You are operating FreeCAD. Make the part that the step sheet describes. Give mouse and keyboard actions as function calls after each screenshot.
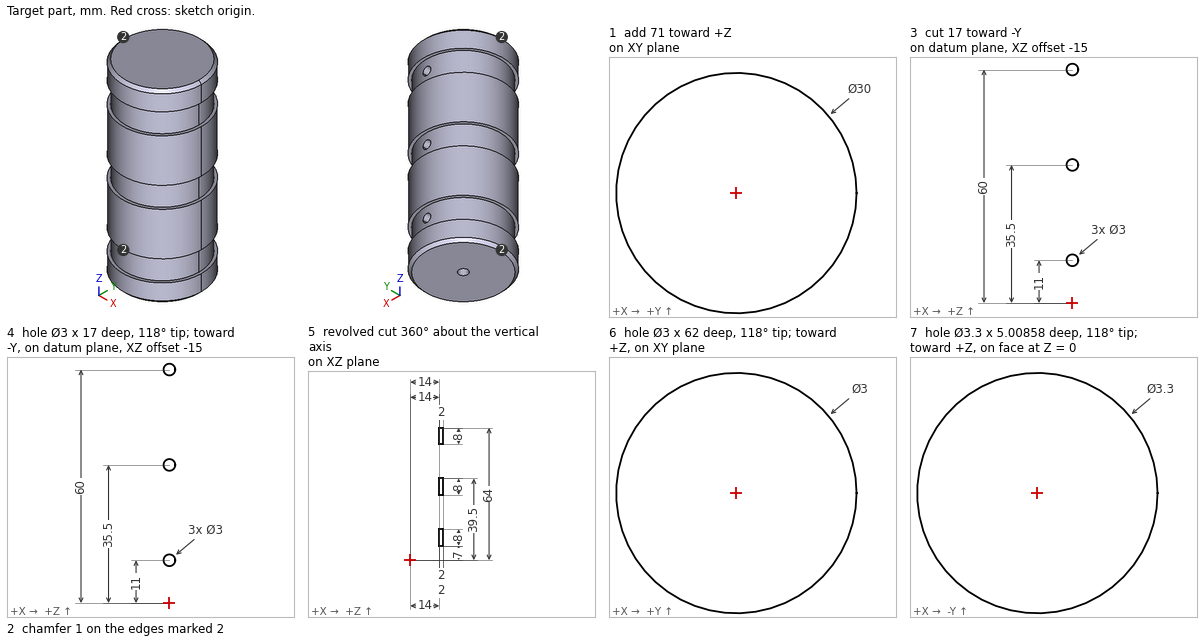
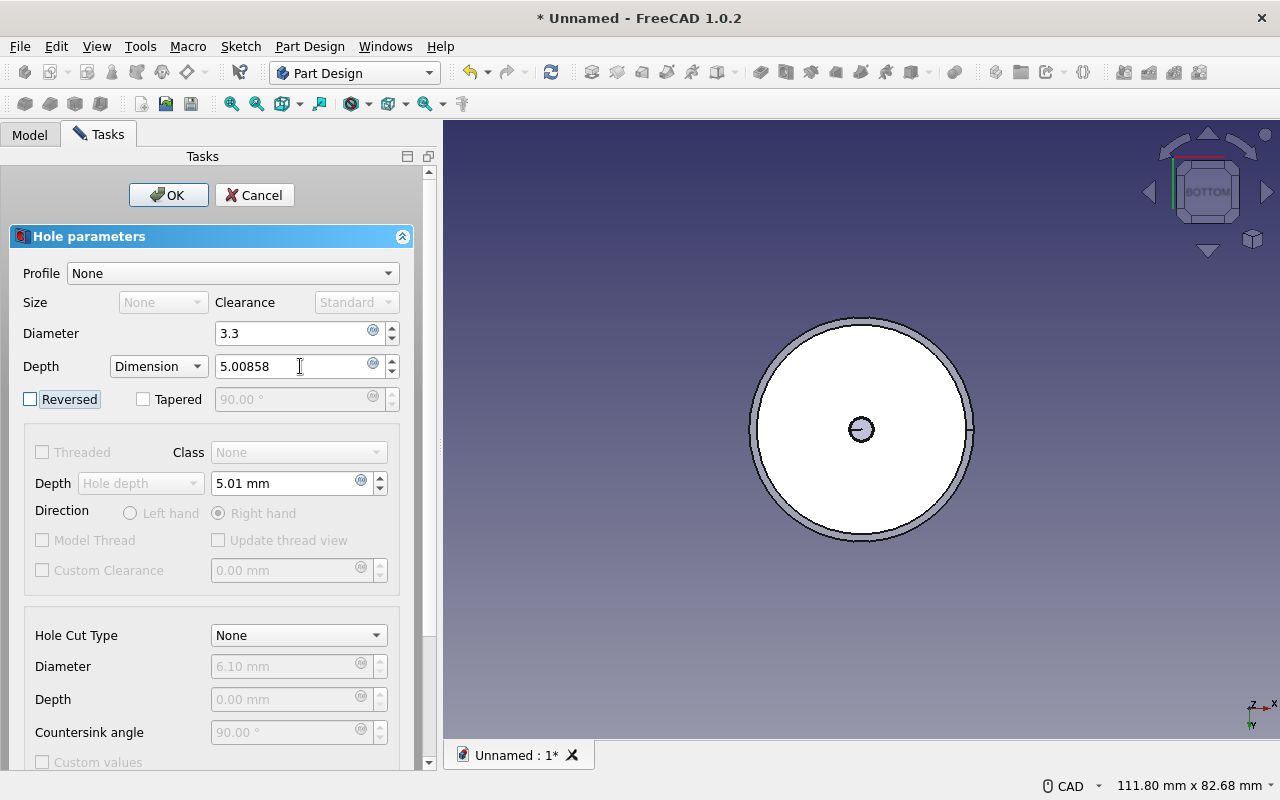
click(169, 195)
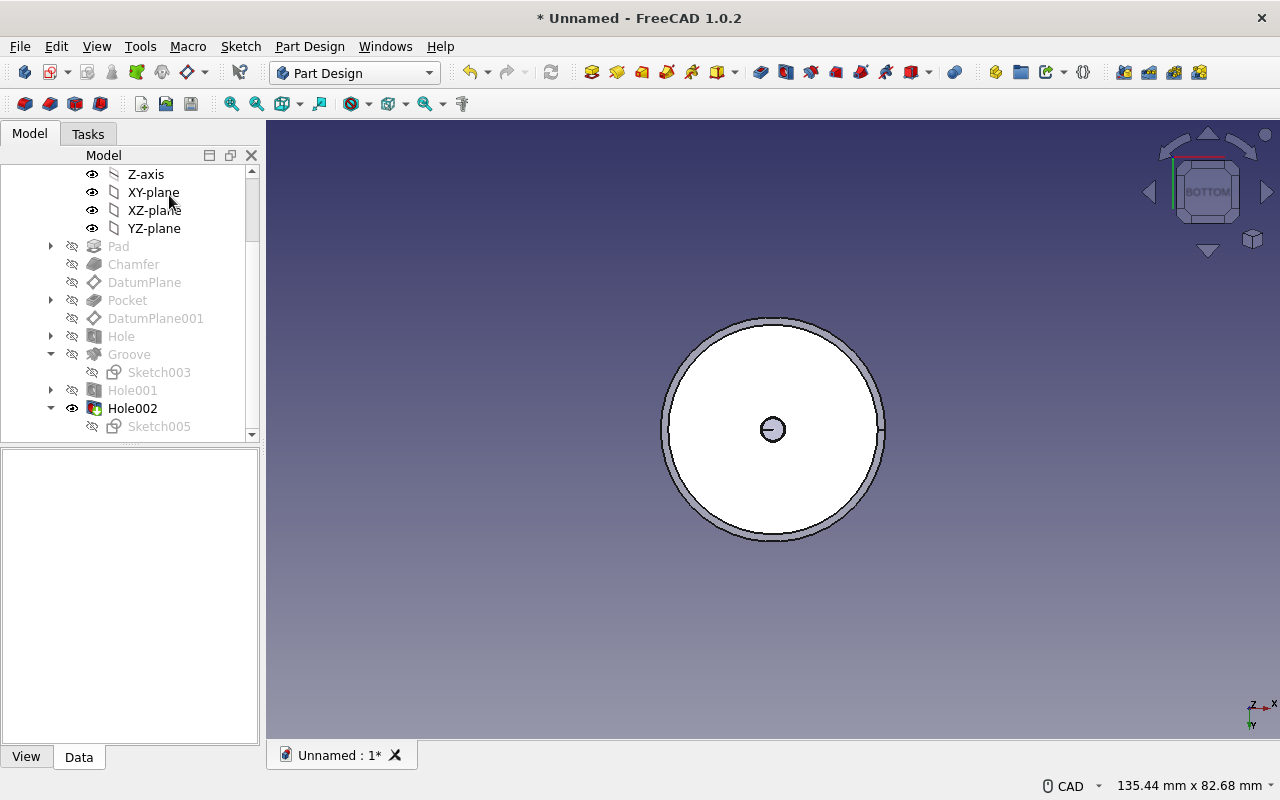
key(0)